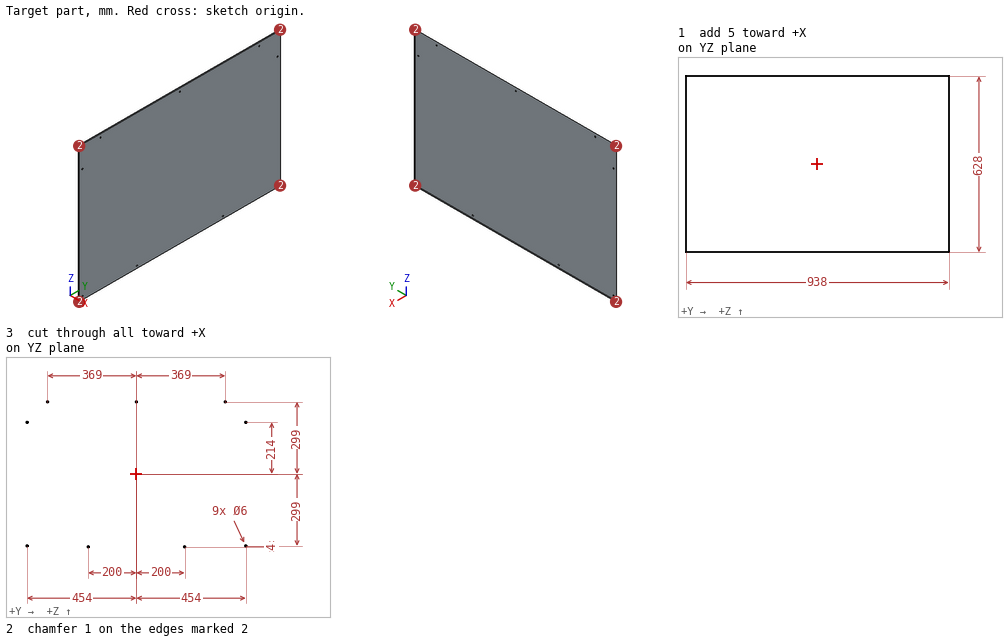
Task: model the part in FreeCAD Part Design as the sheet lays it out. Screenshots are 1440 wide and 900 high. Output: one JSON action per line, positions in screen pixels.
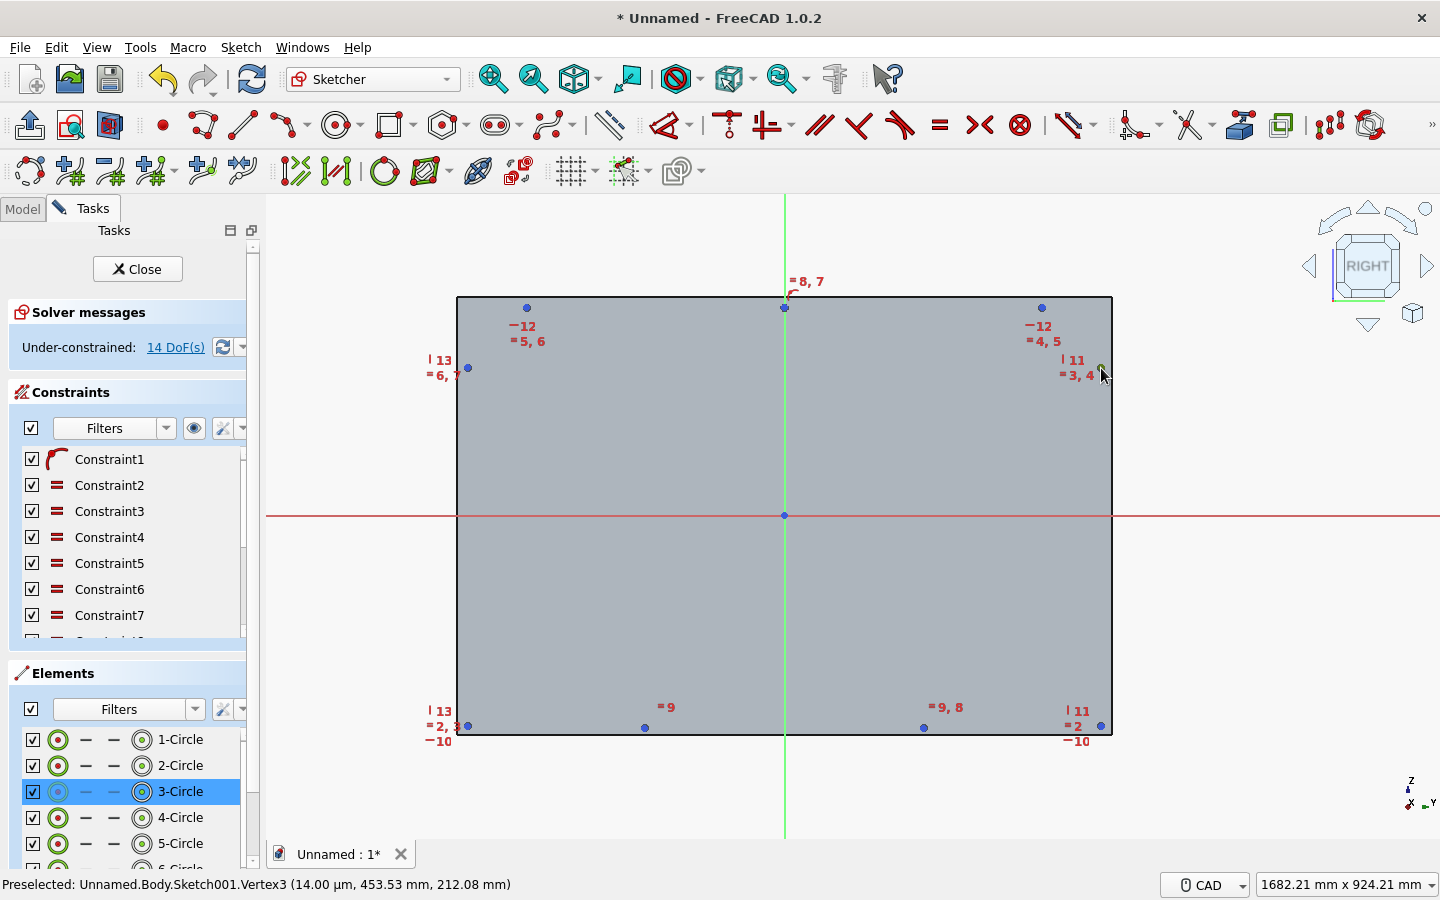
{"action": "left_click", "coordinate": [468, 368]}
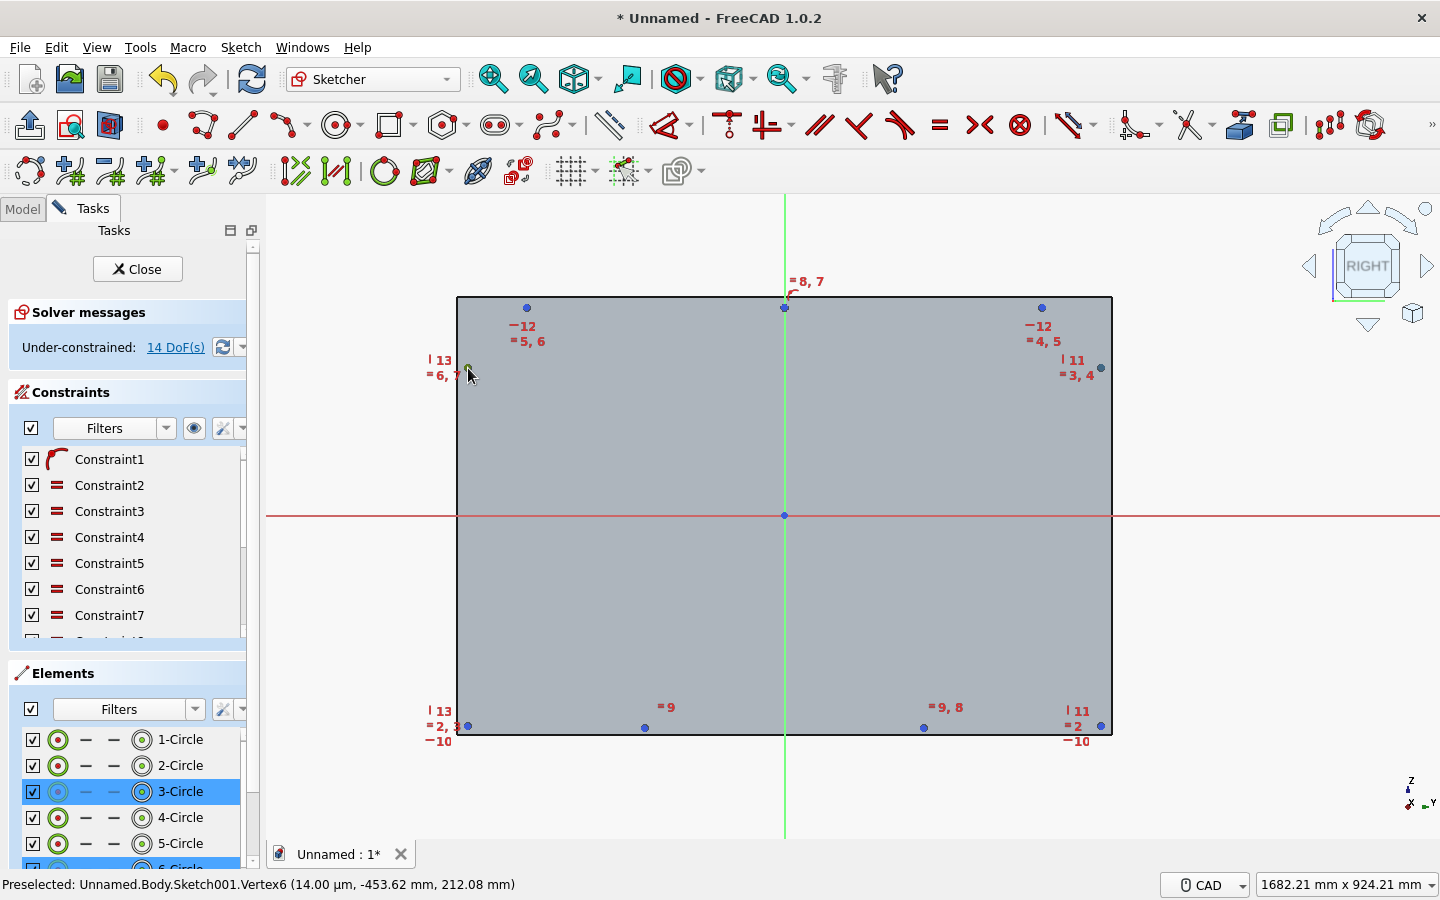
{"action": "key", "text": "h"}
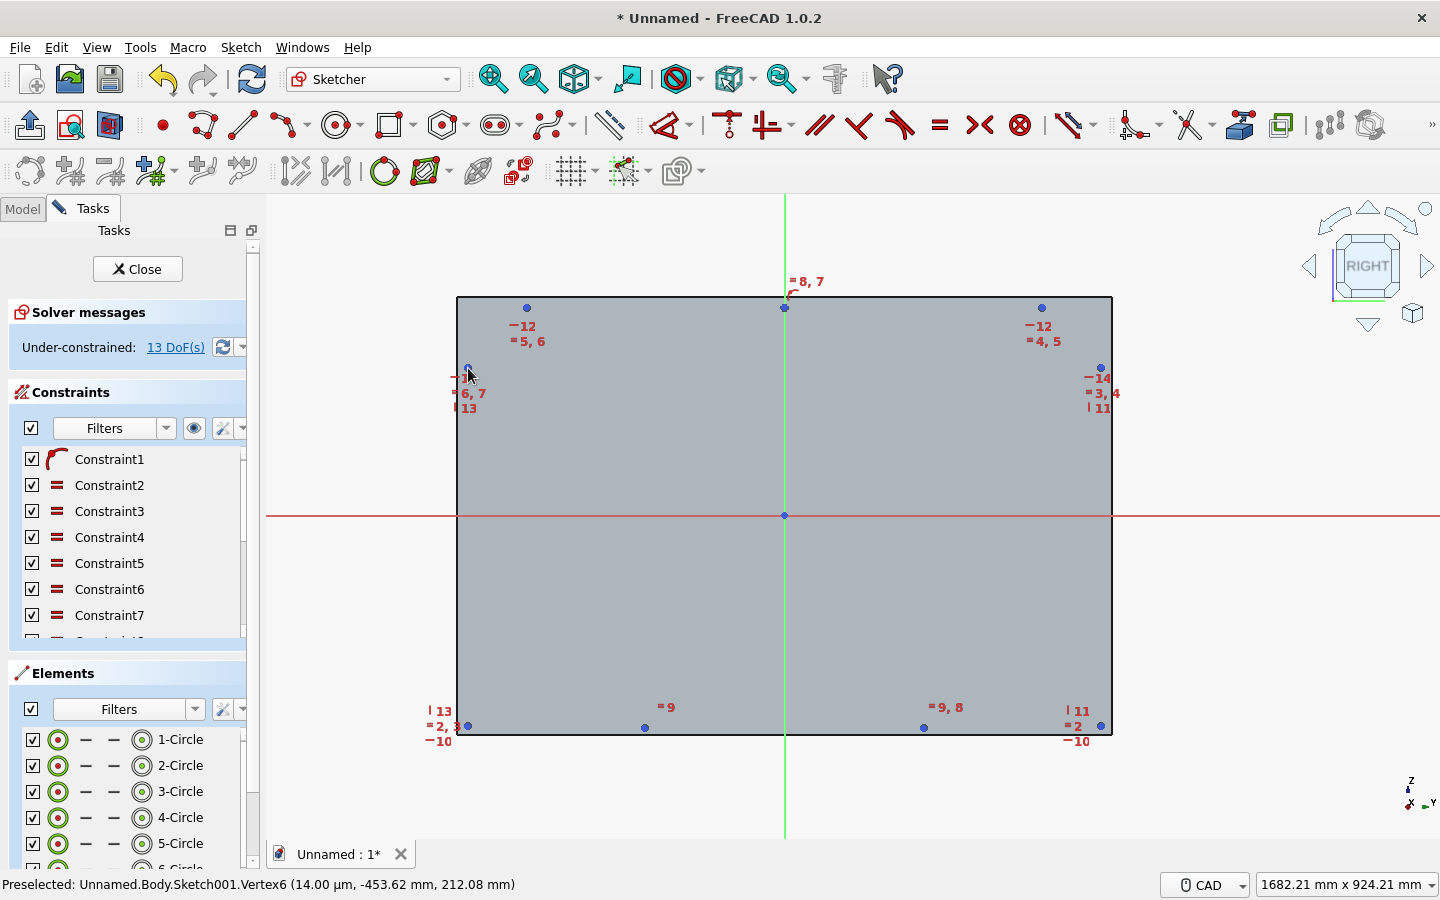
{"action": "left_click", "coordinate": [1042, 308]}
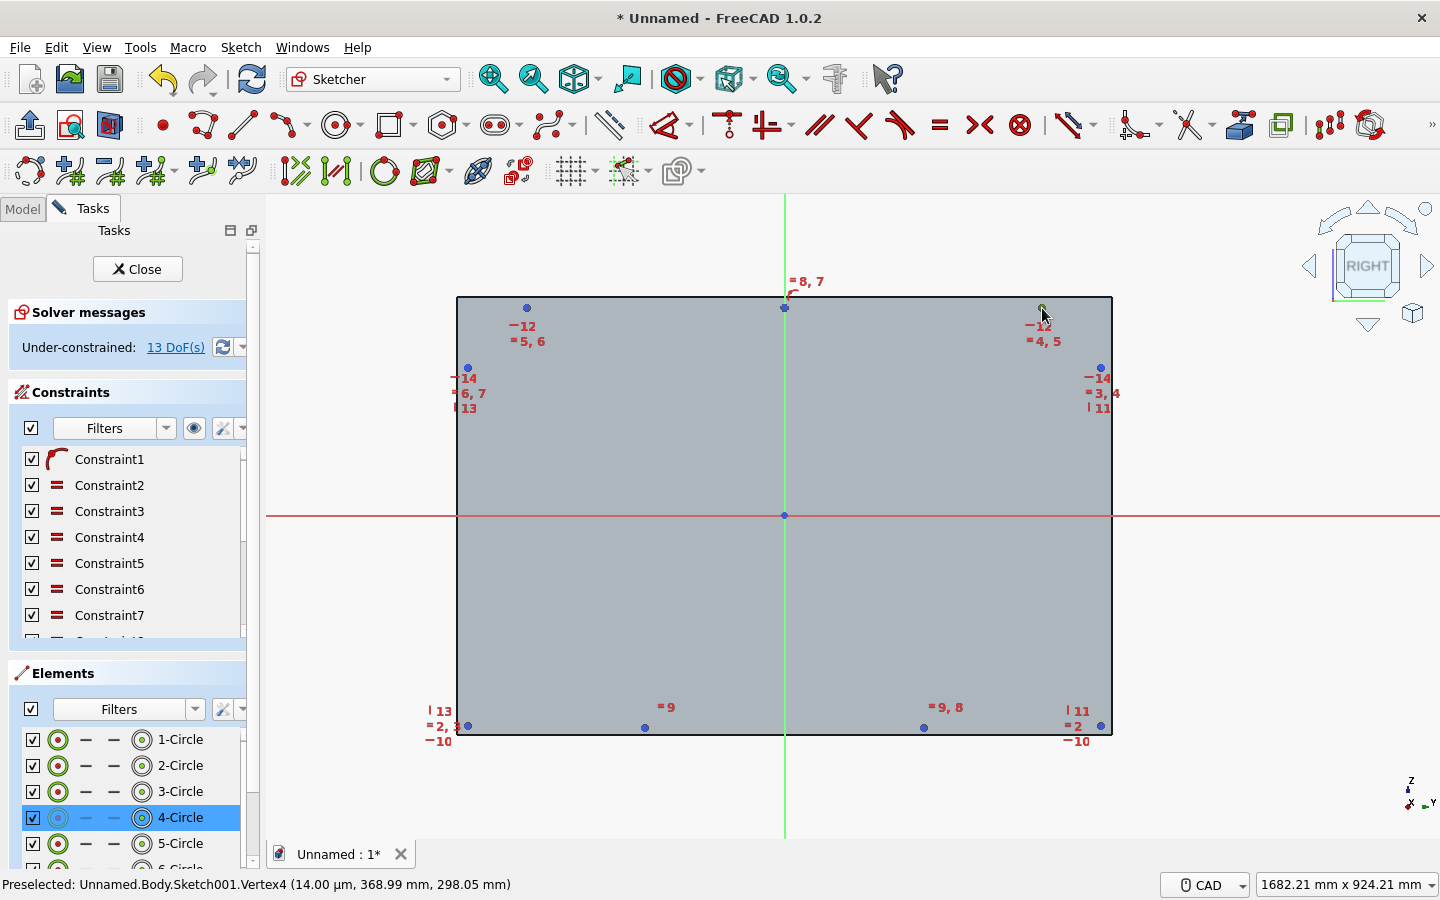
{"action": "left_click", "coordinate": [785, 308]}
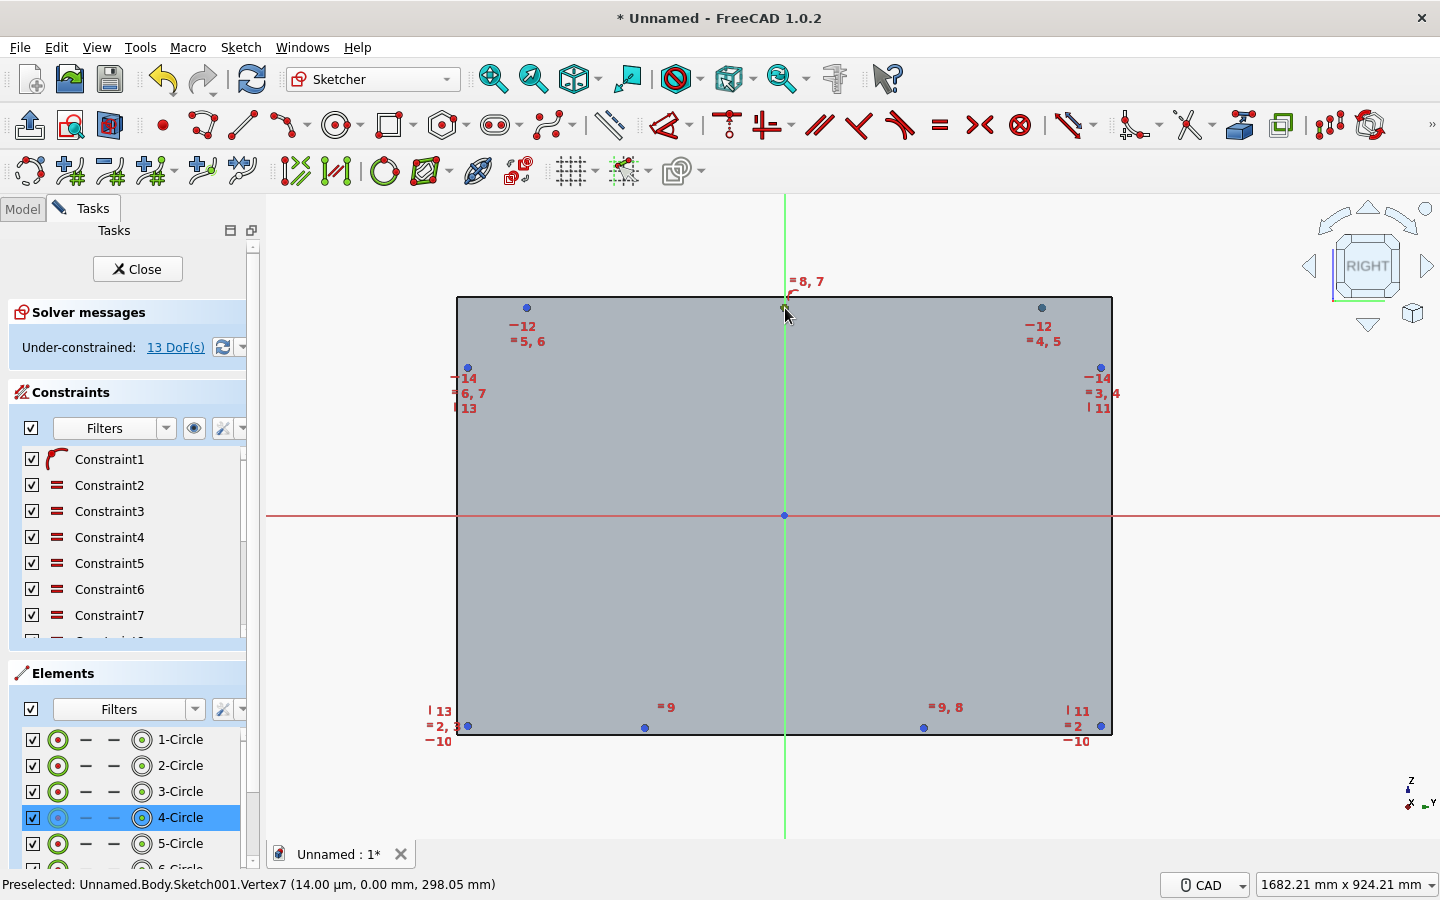
{"action": "key", "text": "h"}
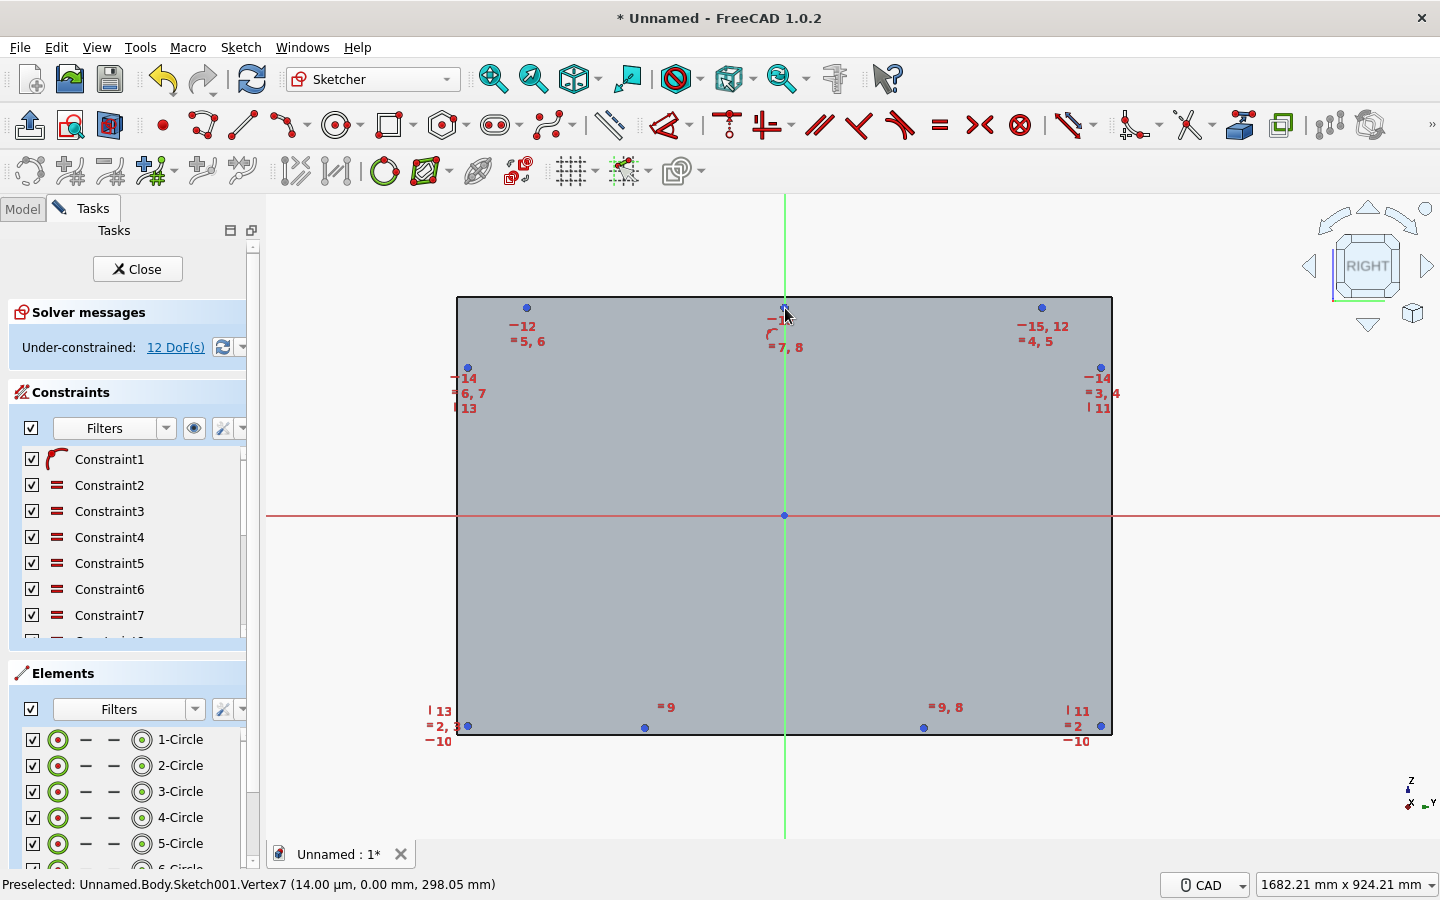
{"action": "left_click", "coordinate": [924, 728]}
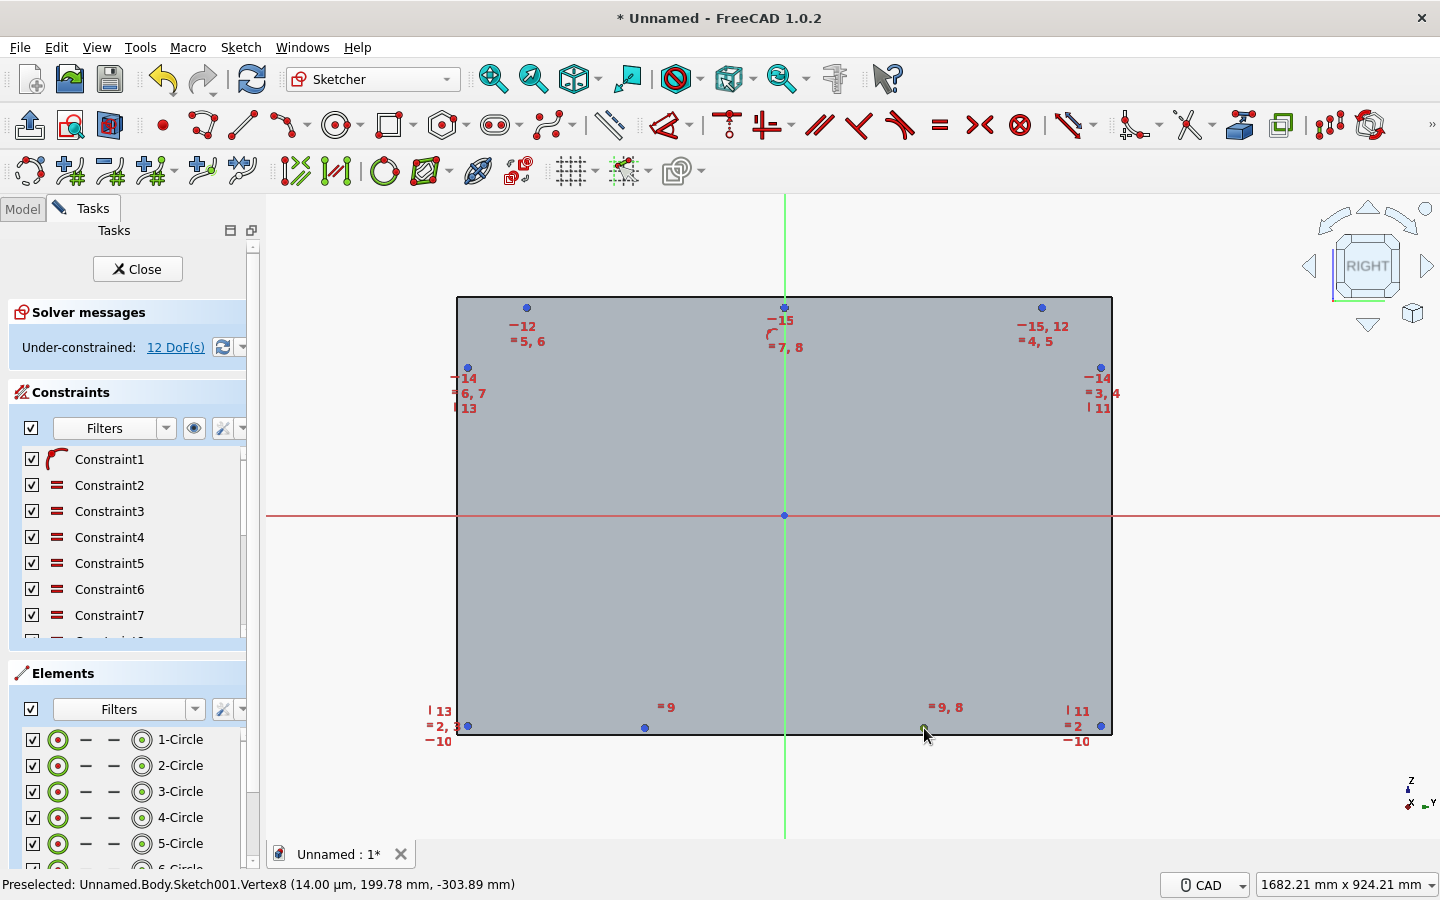
{"action": "left_click", "coordinate": [645, 728]}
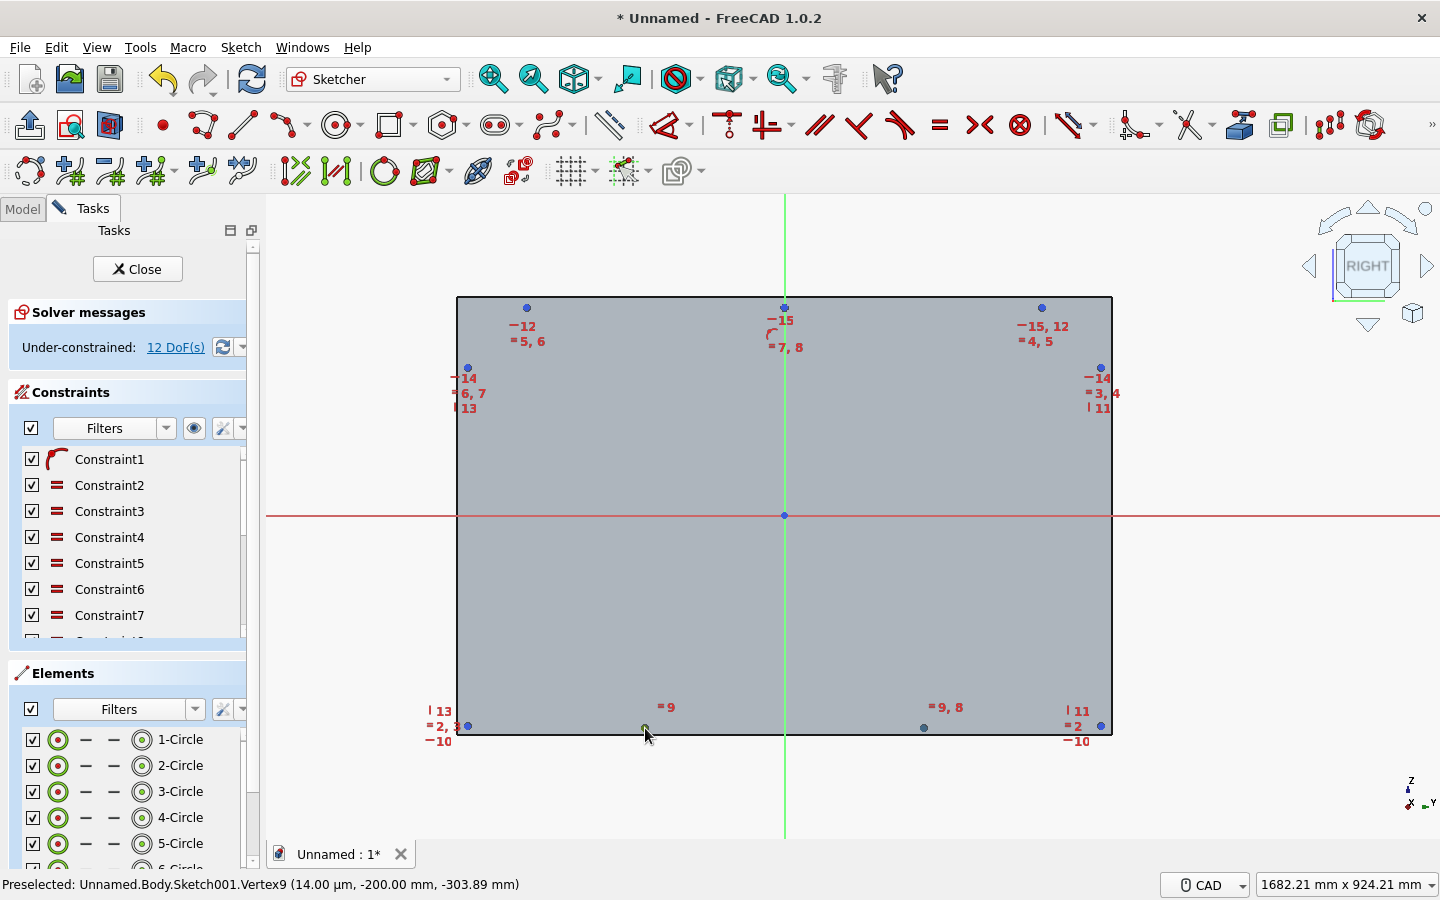
{"action": "left_click", "coordinate": [794, 126]}